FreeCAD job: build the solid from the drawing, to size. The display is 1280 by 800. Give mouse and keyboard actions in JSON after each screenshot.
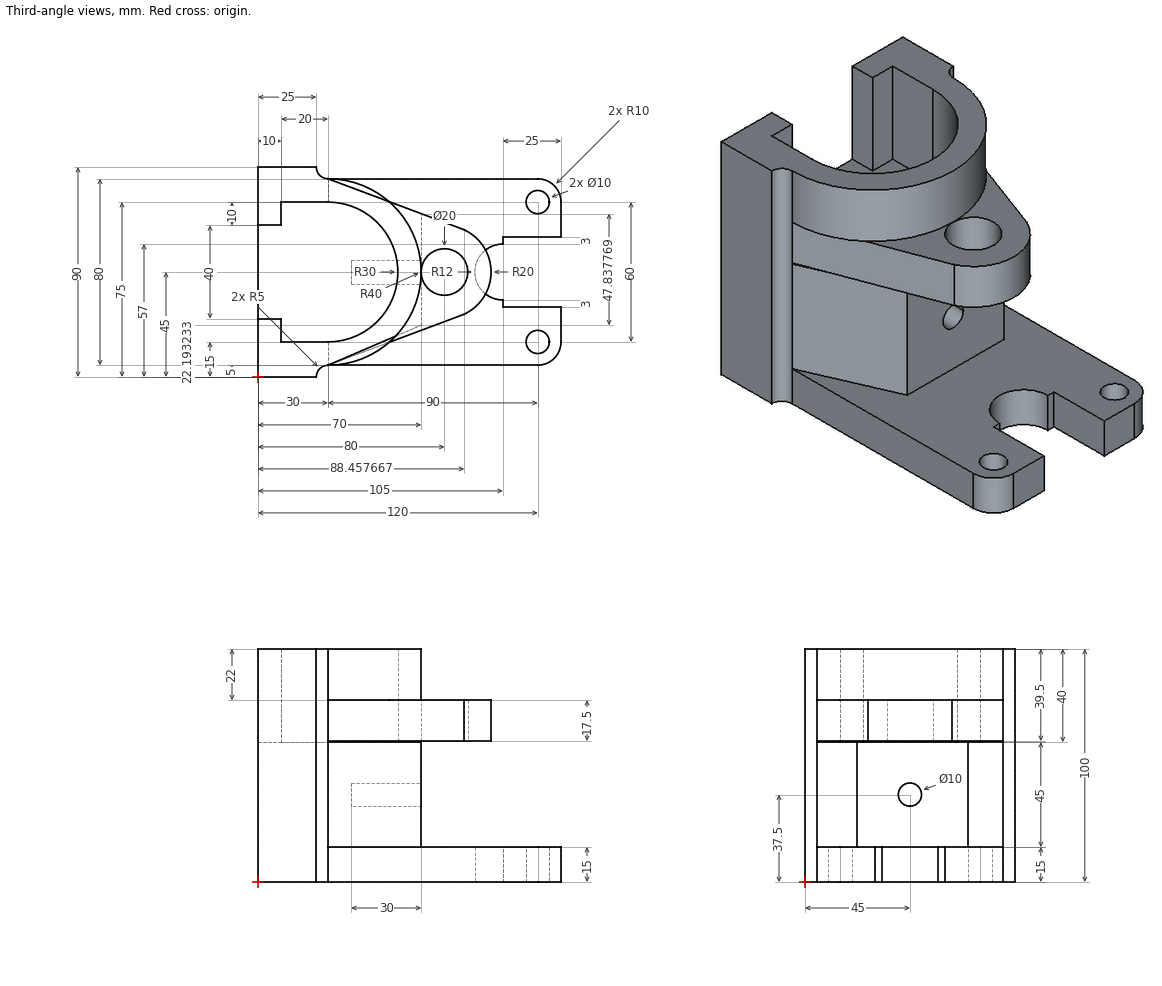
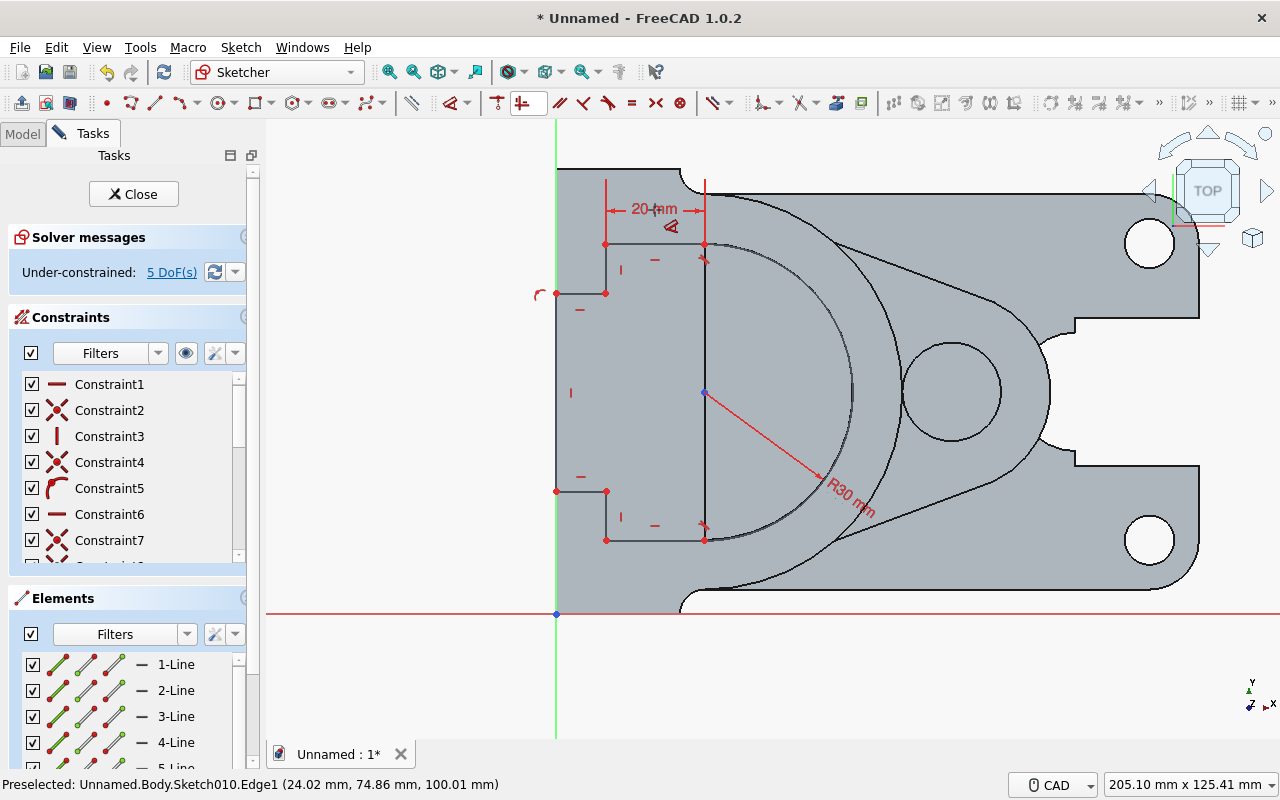
{"action": "left_click", "coordinate": [606, 259]}
{"action": "left_click", "coordinate": [572, 269]}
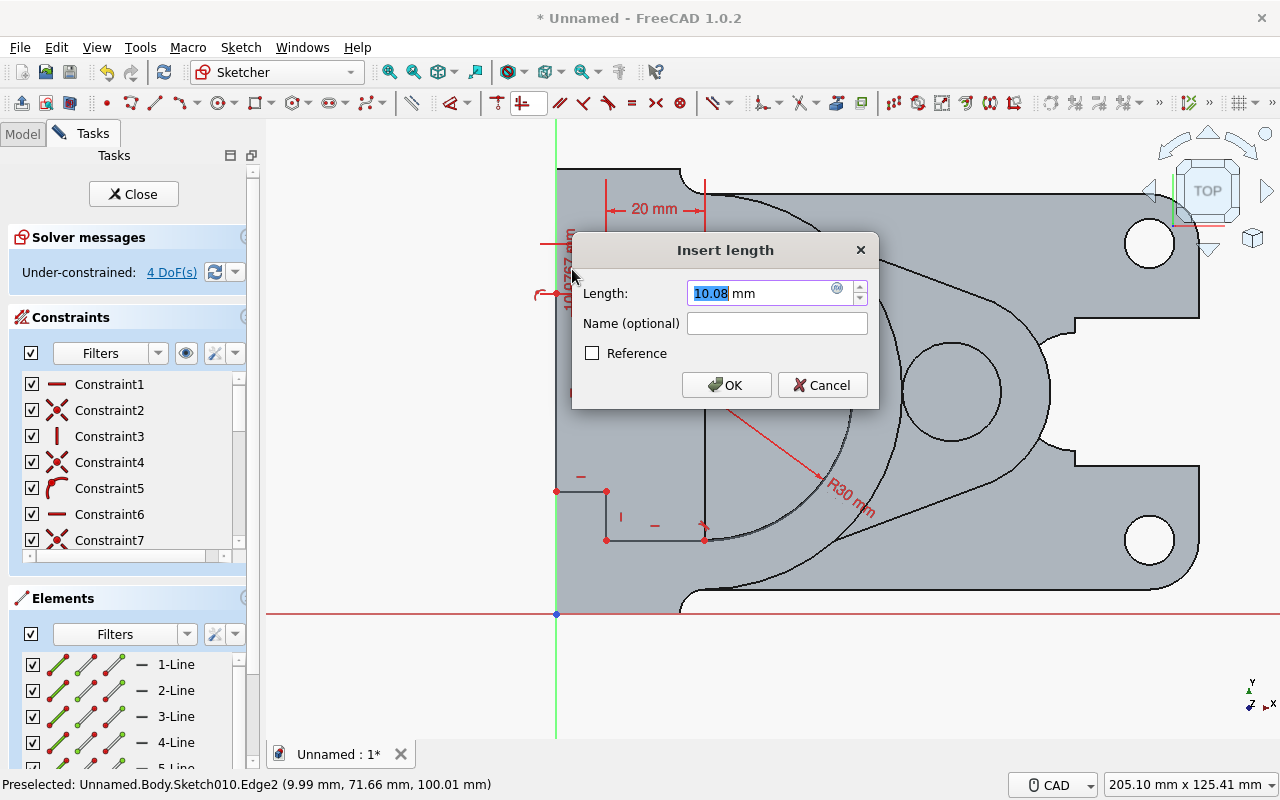
{"action": "type", "text": "10"}
{"action": "key", "text": "Return"}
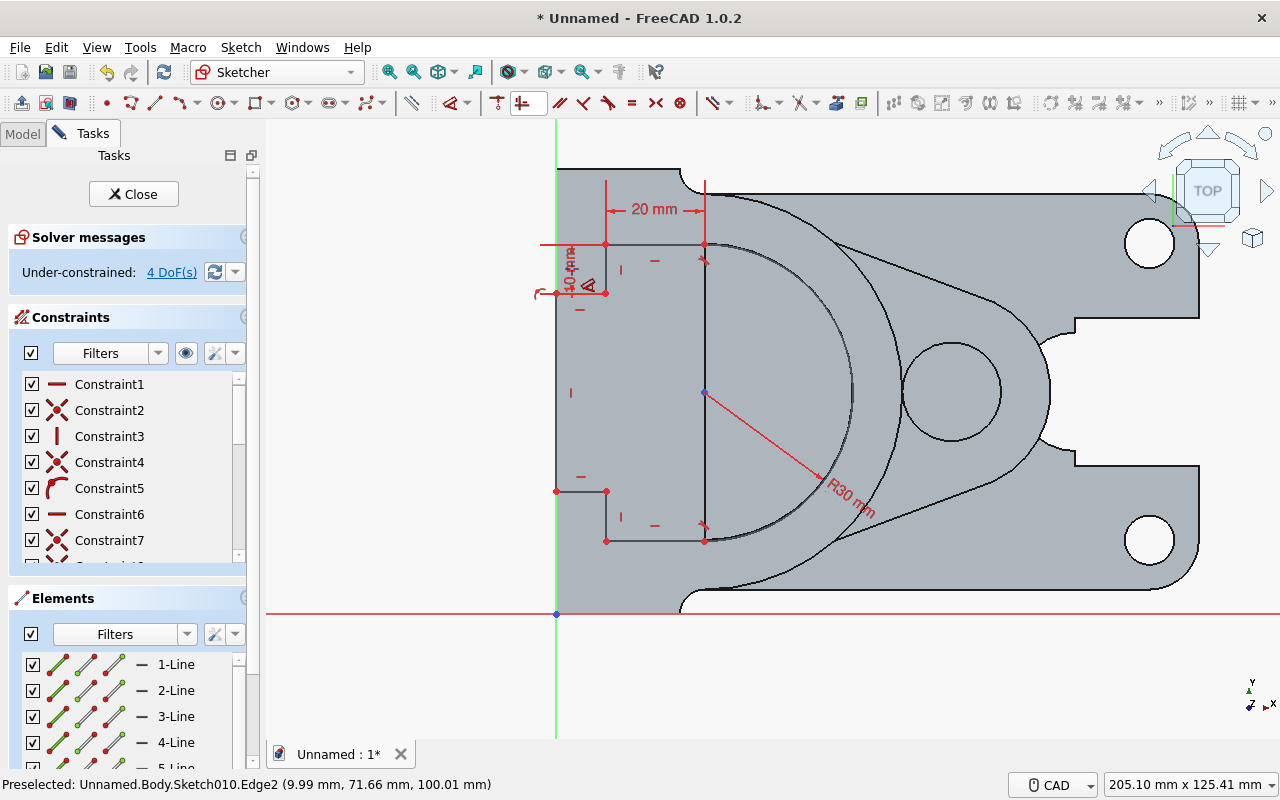
{"action": "left_click", "coordinate": [591, 294]}
{"action": "left_click", "coordinate": [581, 328]}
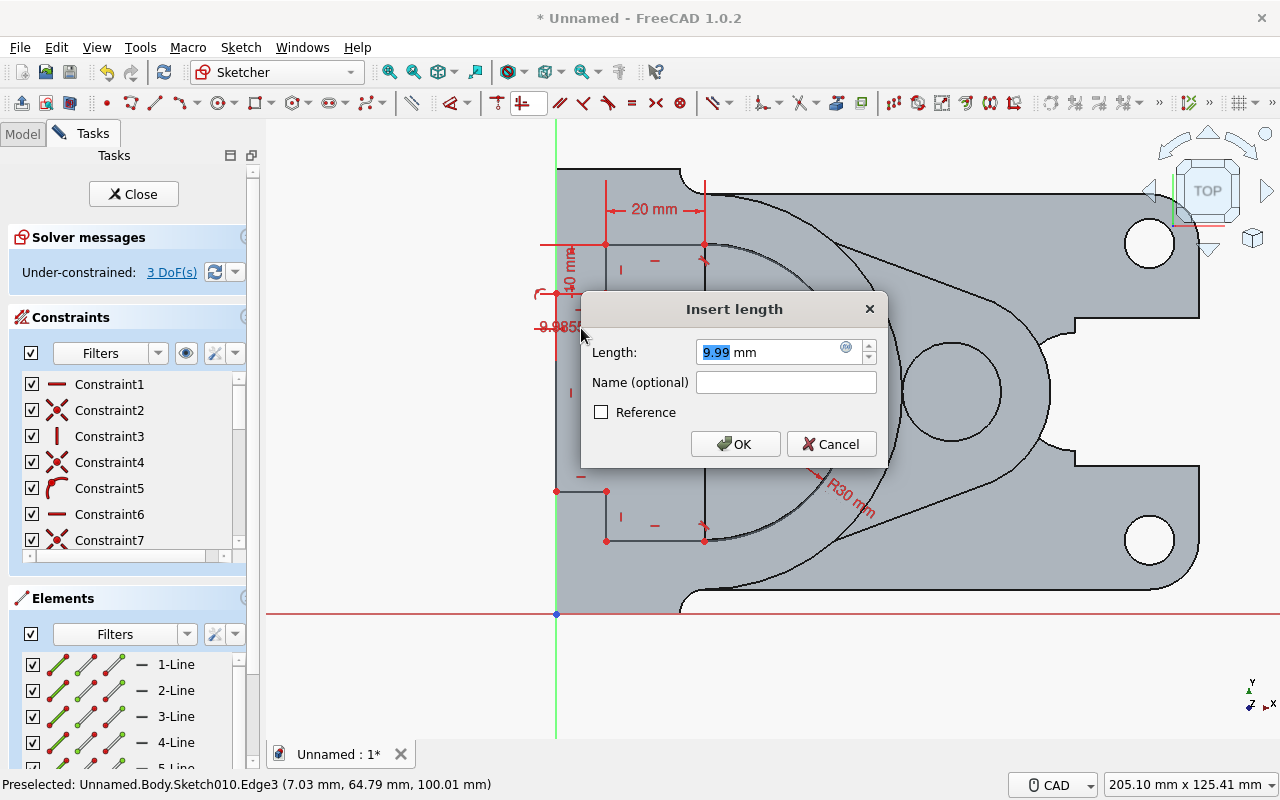
{"action": "type", "text": "10"}
{"action": "key", "text": "Return"}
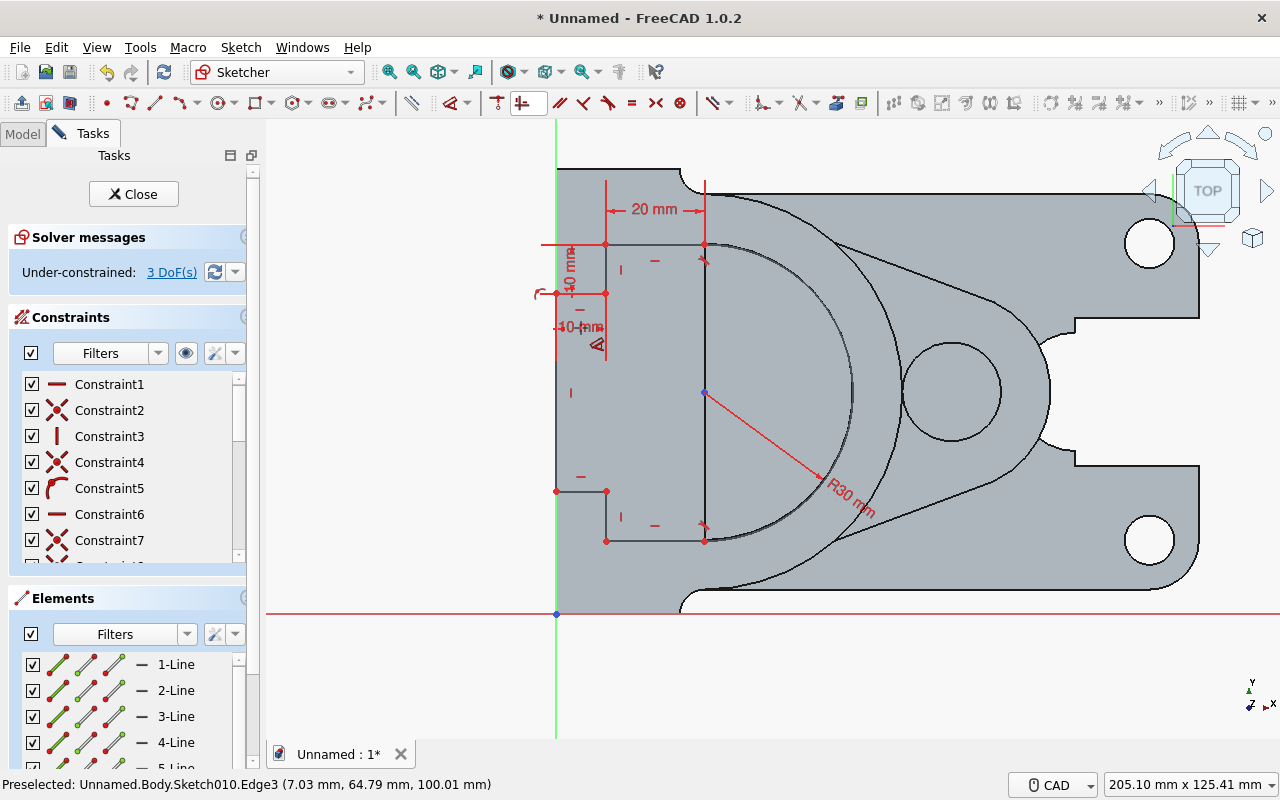
{"action": "left_click", "coordinate": [556, 353]}
{"action": "left_click", "coordinate": [522, 393]}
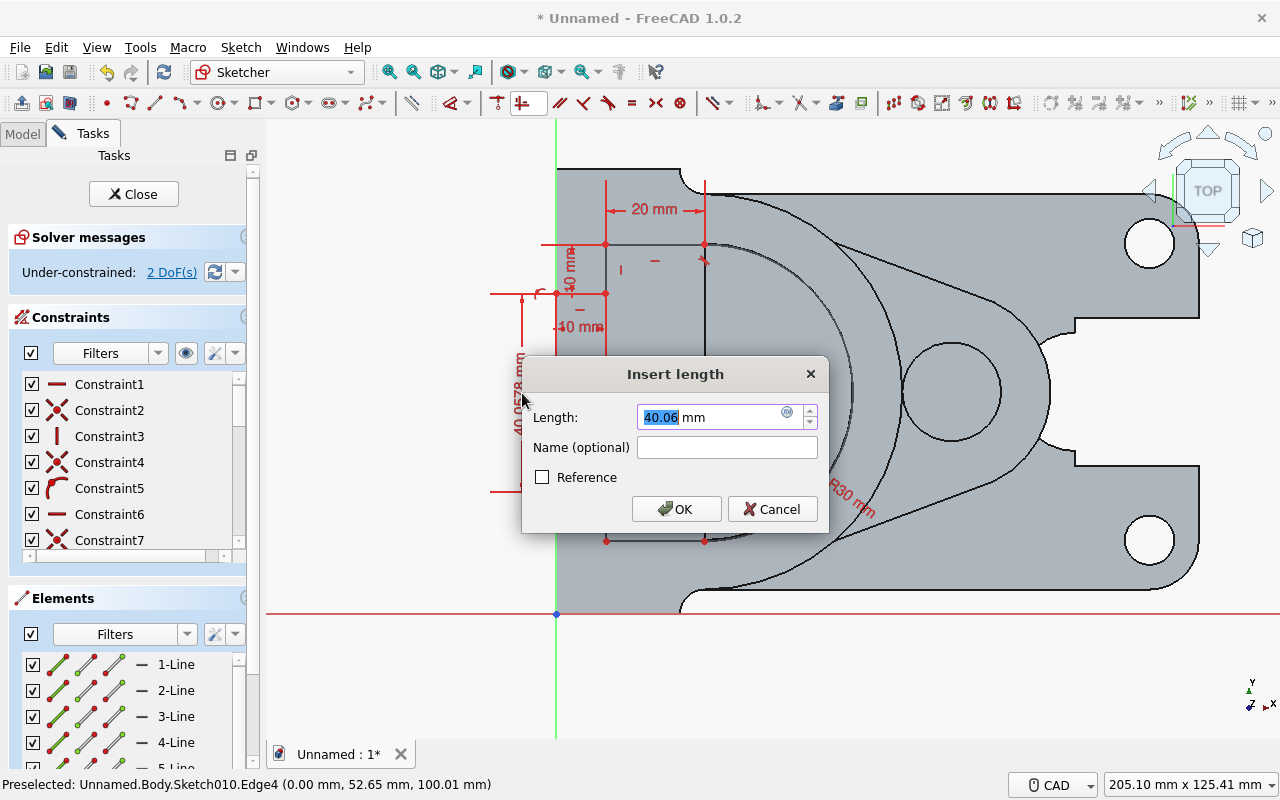
{"action": "type", "text": "40"}
{"action": "key", "text": "Return"}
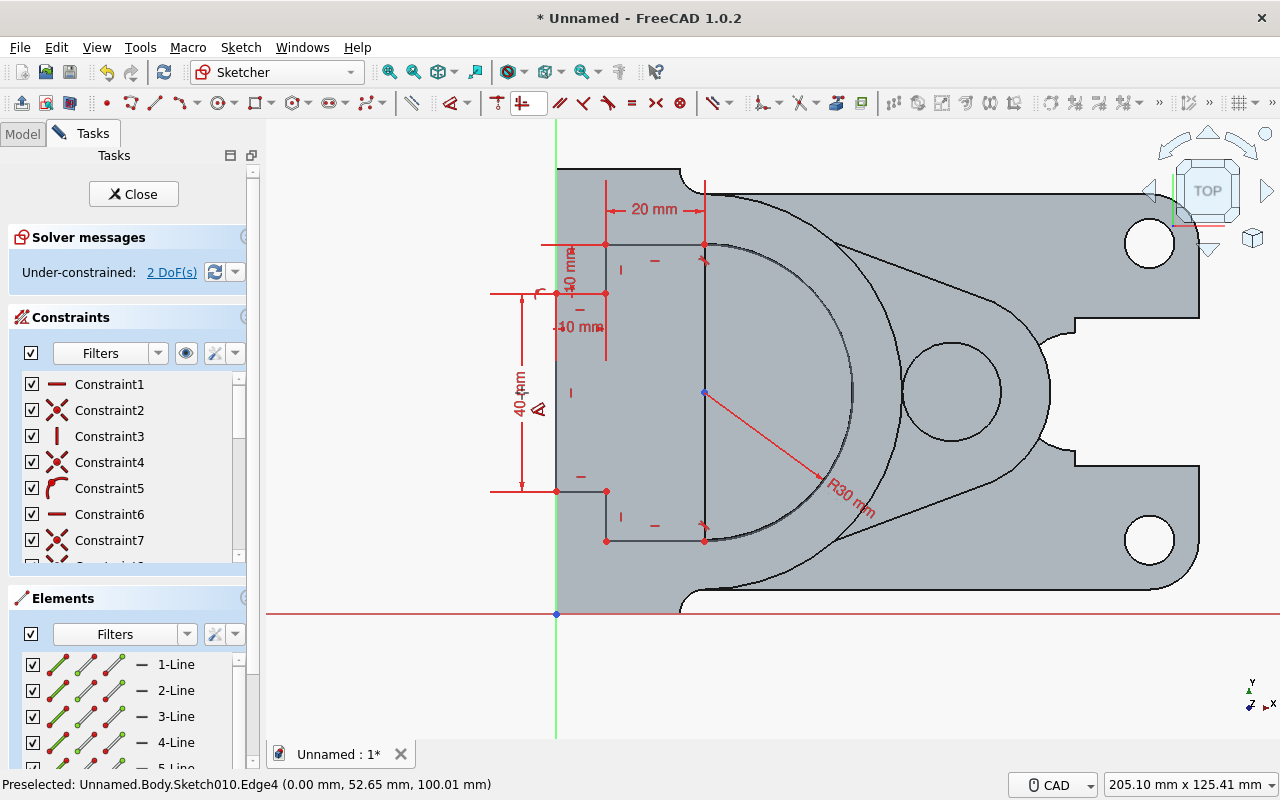
{"action": "left_click", "coordinate": [571, 492]}
{"action": "left_click", "coordinate": [581, 526]}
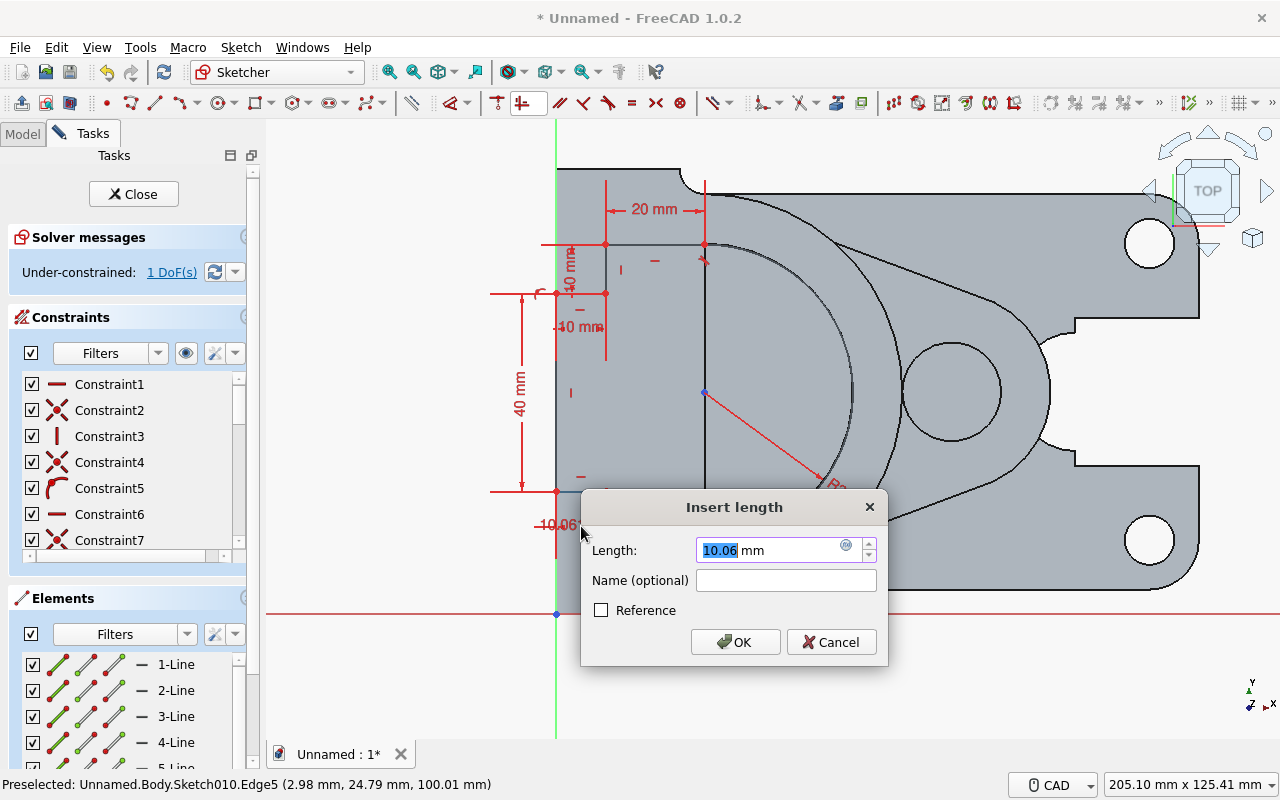
{"action": "type", "text": "10"}
{"action": "key", "text": "Return"}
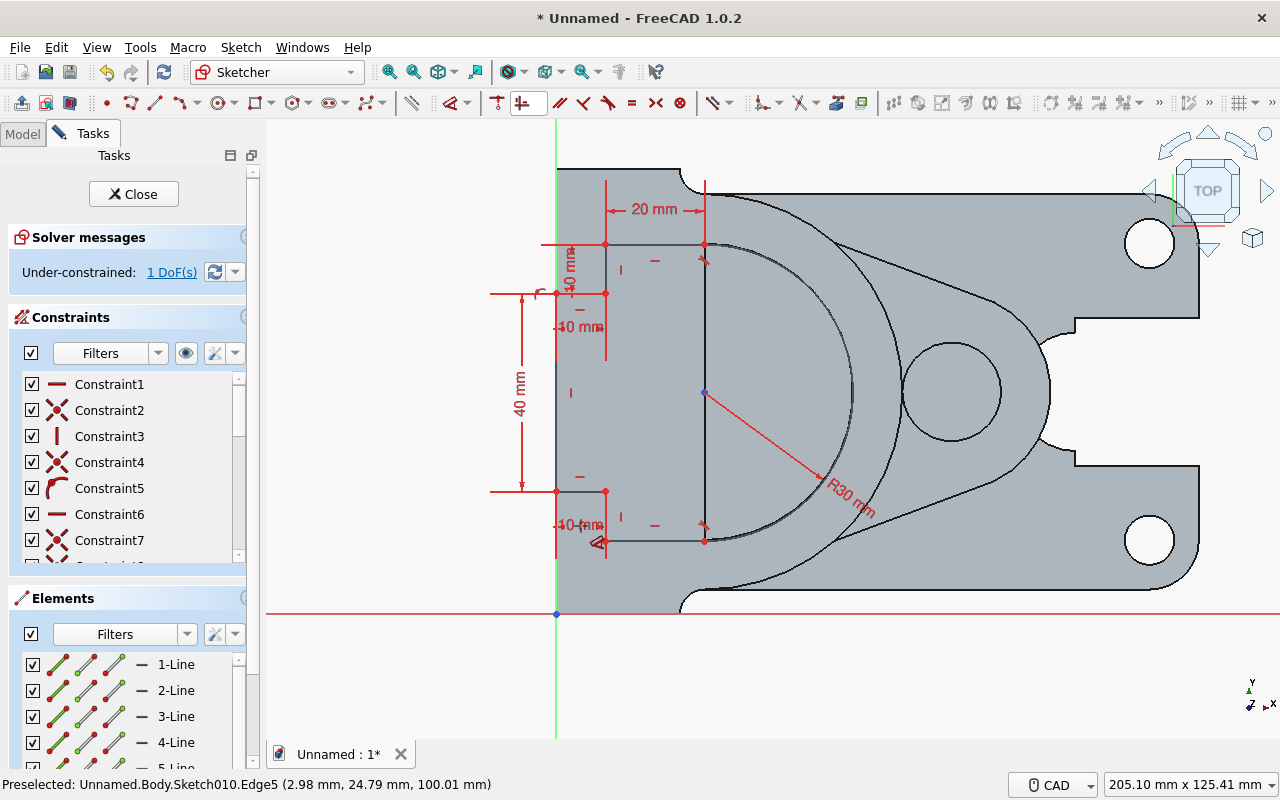
{"action": "left_click", "coordinate": [705, 245]}
{"action": "left_click", "coordinate": [522, 429]}